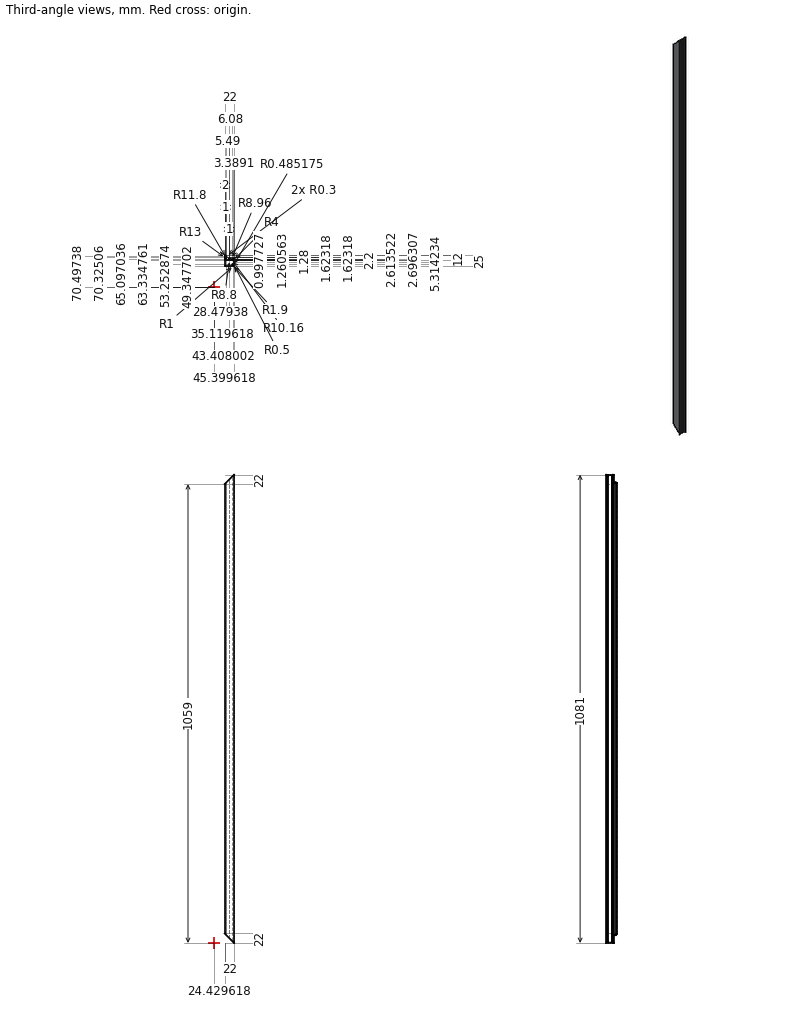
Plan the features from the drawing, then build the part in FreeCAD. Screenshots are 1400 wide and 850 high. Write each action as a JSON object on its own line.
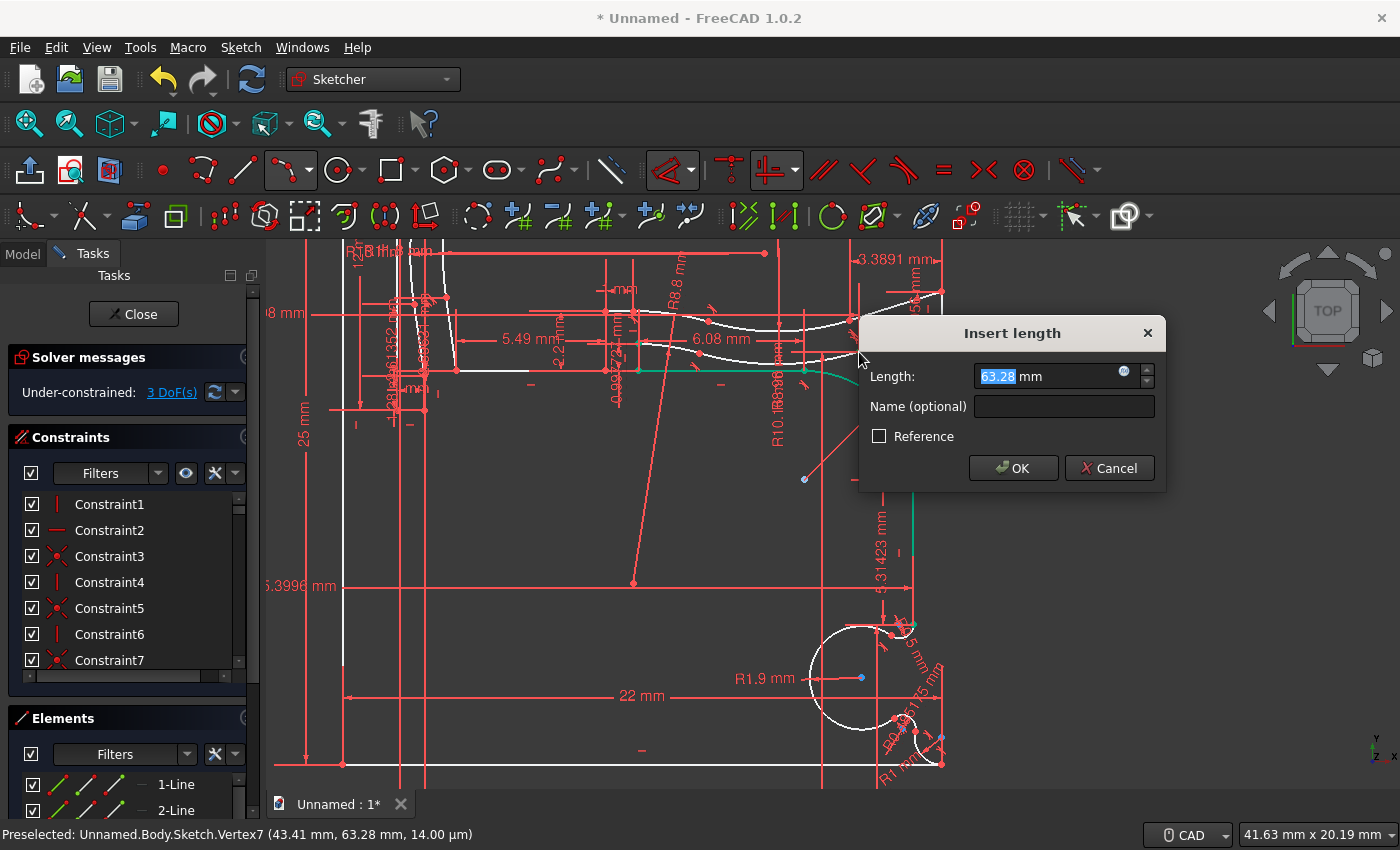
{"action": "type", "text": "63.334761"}
{"action": "key", "text": "Return"}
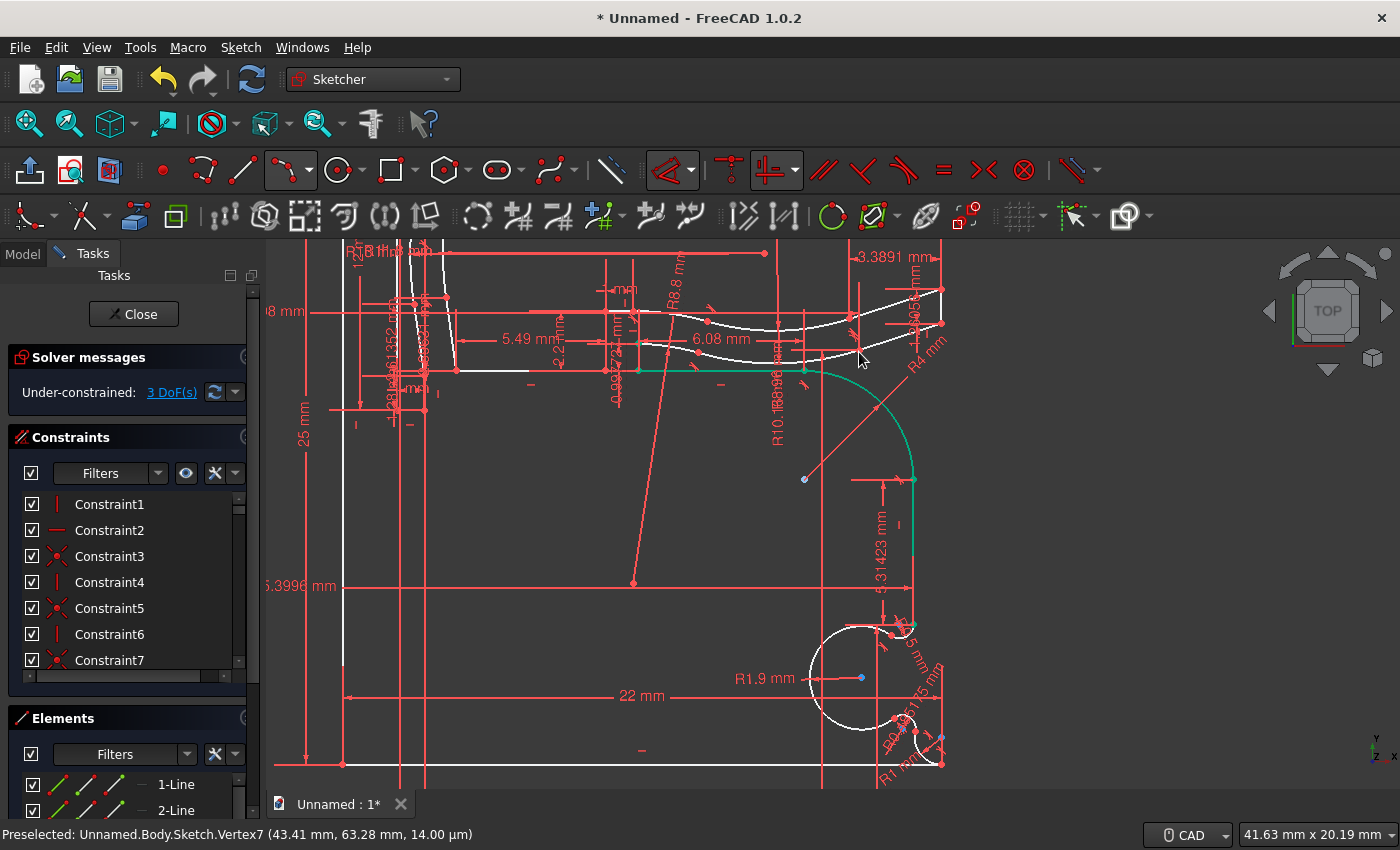
{"action": "left_click", "coordinate": [633, 311]}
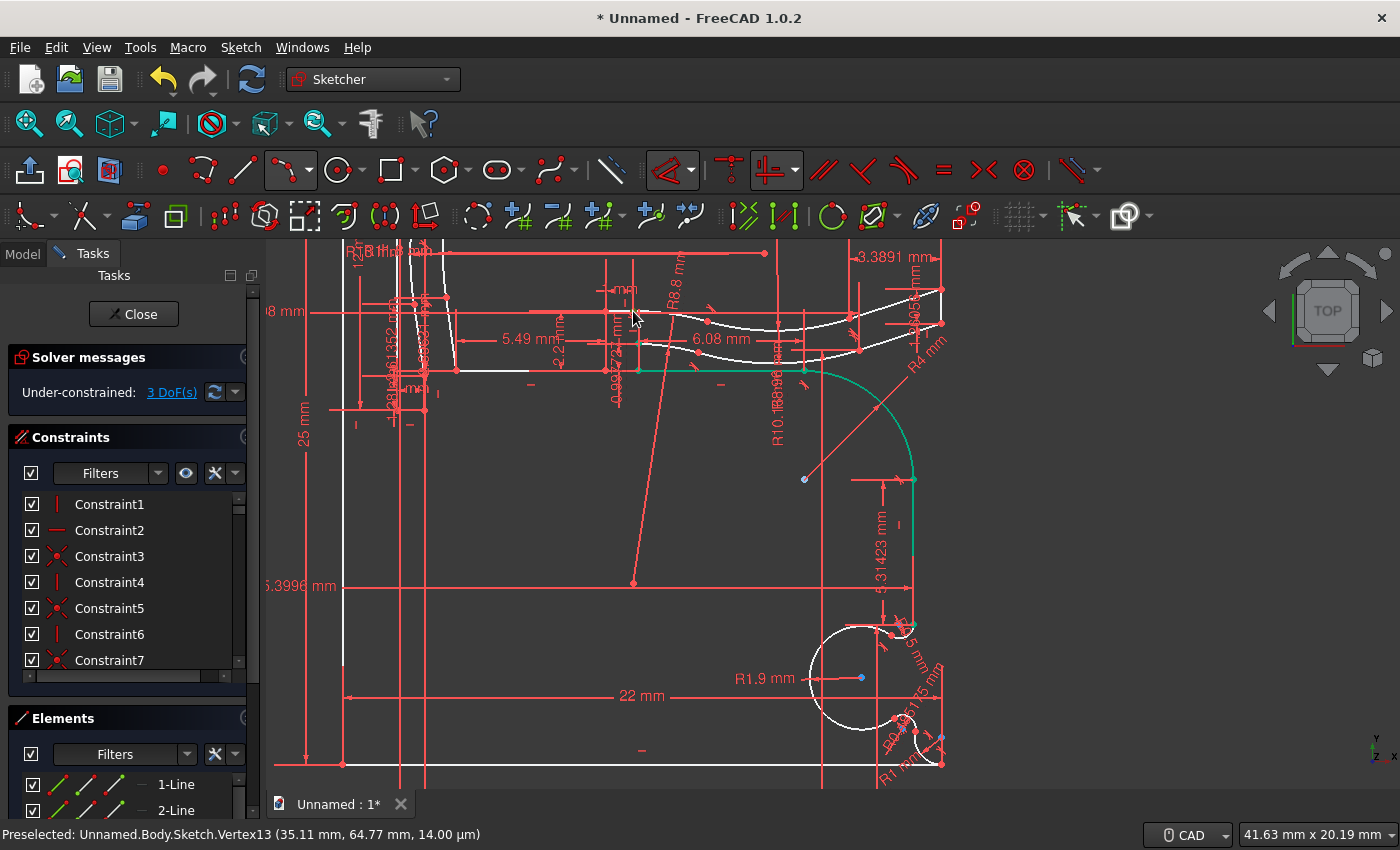
{"action": "left_click", "coordinate": [694, 170]}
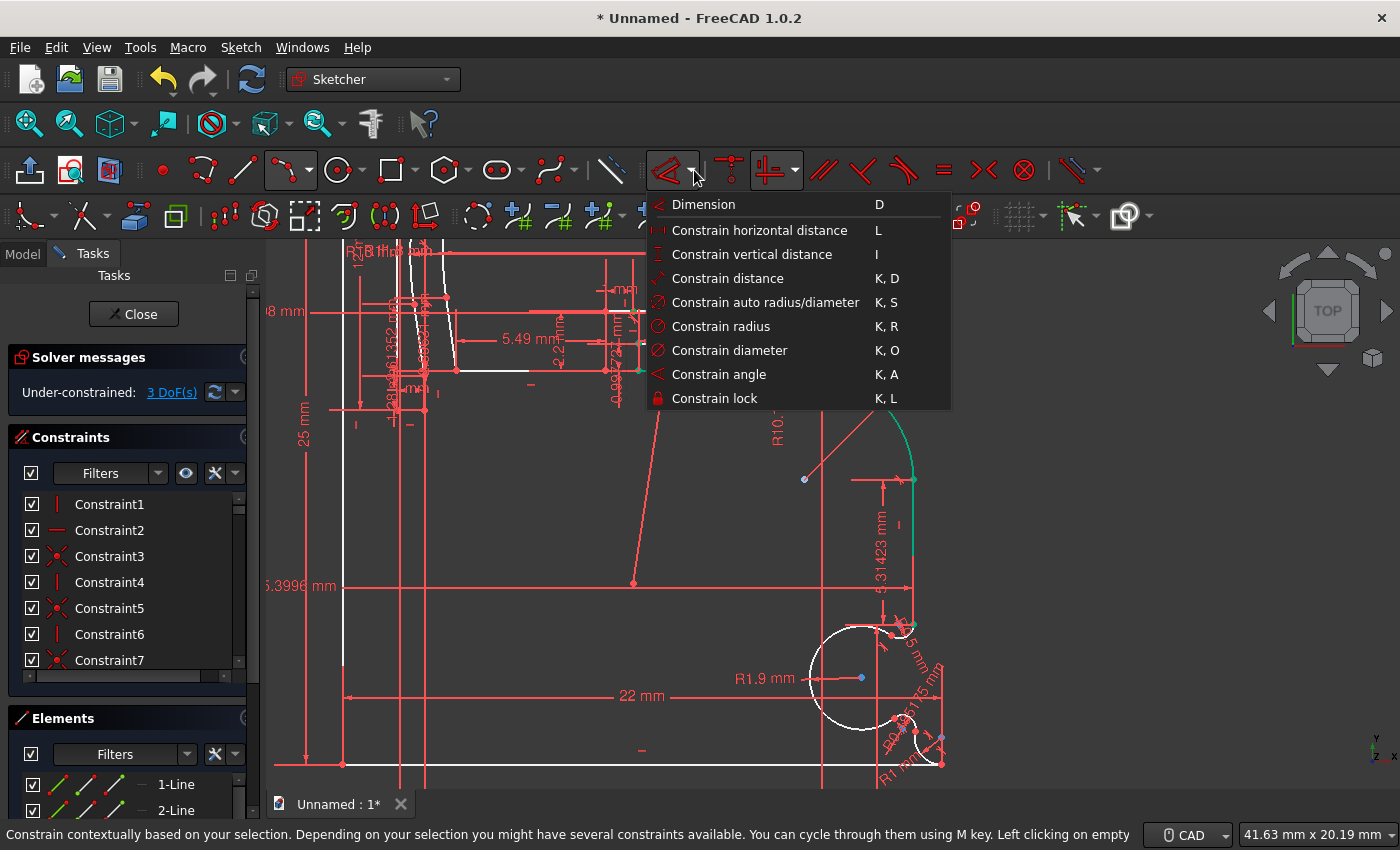
{"action": "left_click", "coordinate": [799, 230]}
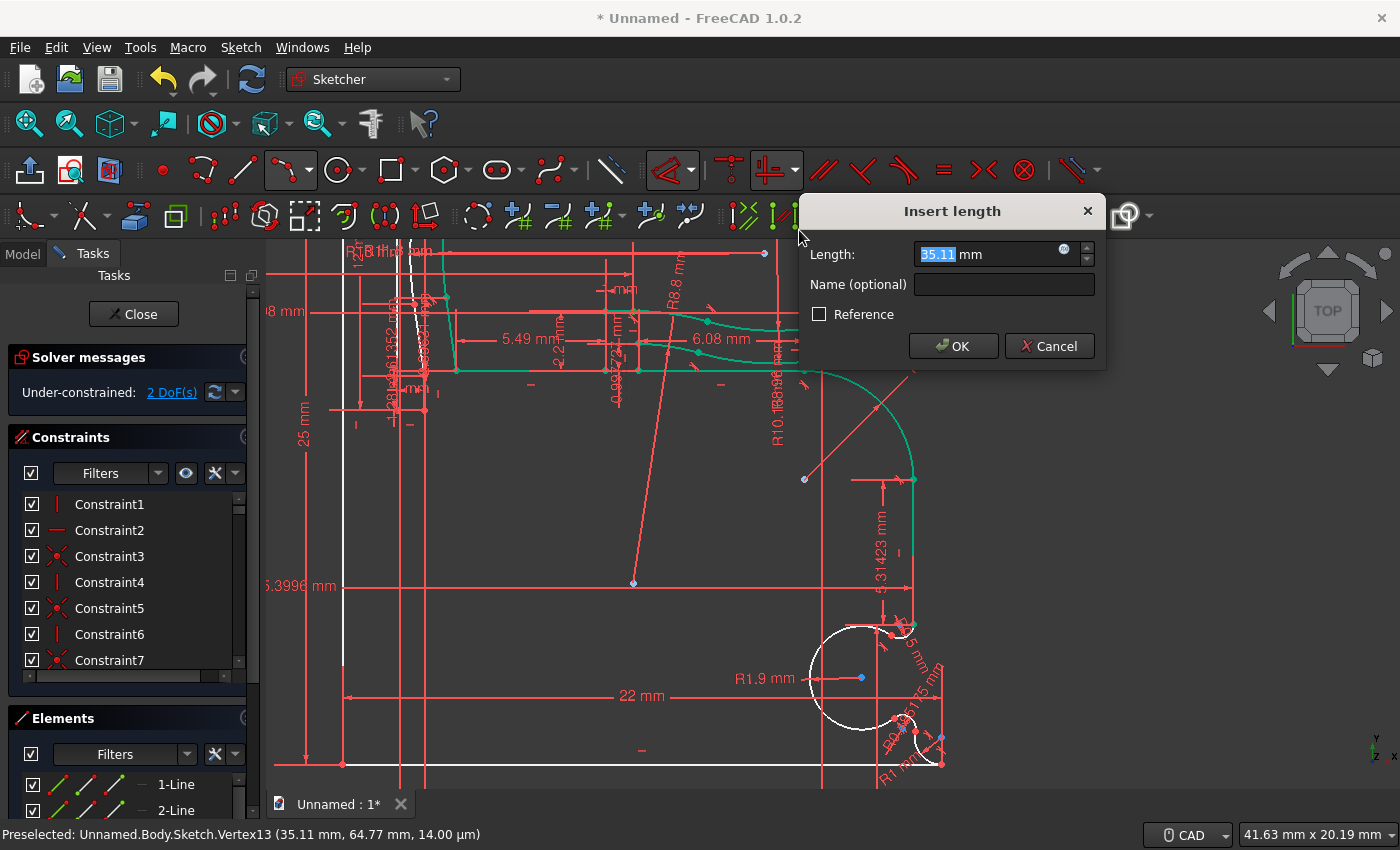
{"action": "type", "text": "35.119618"}
{"action": "key", "text": "Return"}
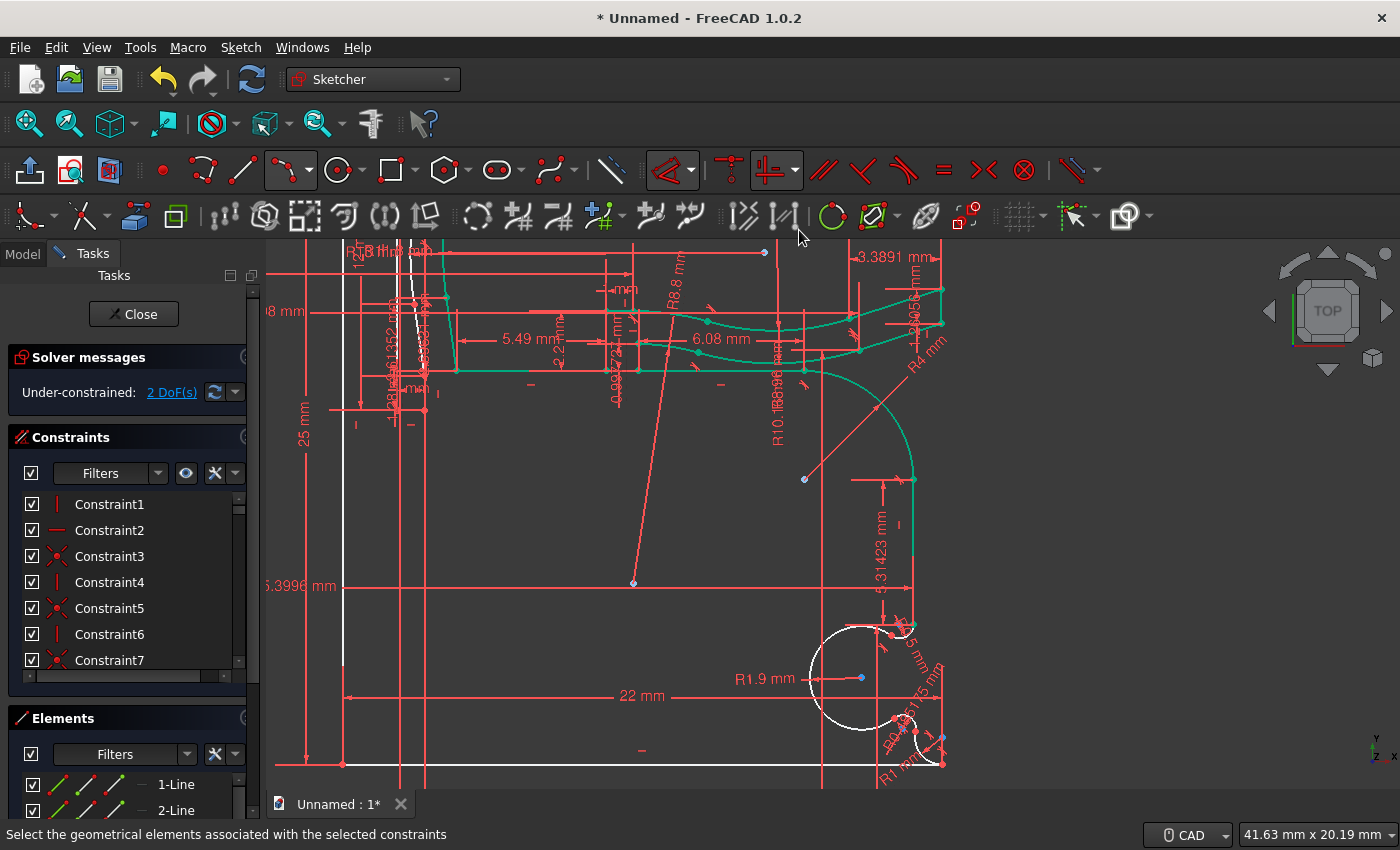
{"action": "left_click", "coordinate": [414, 304]}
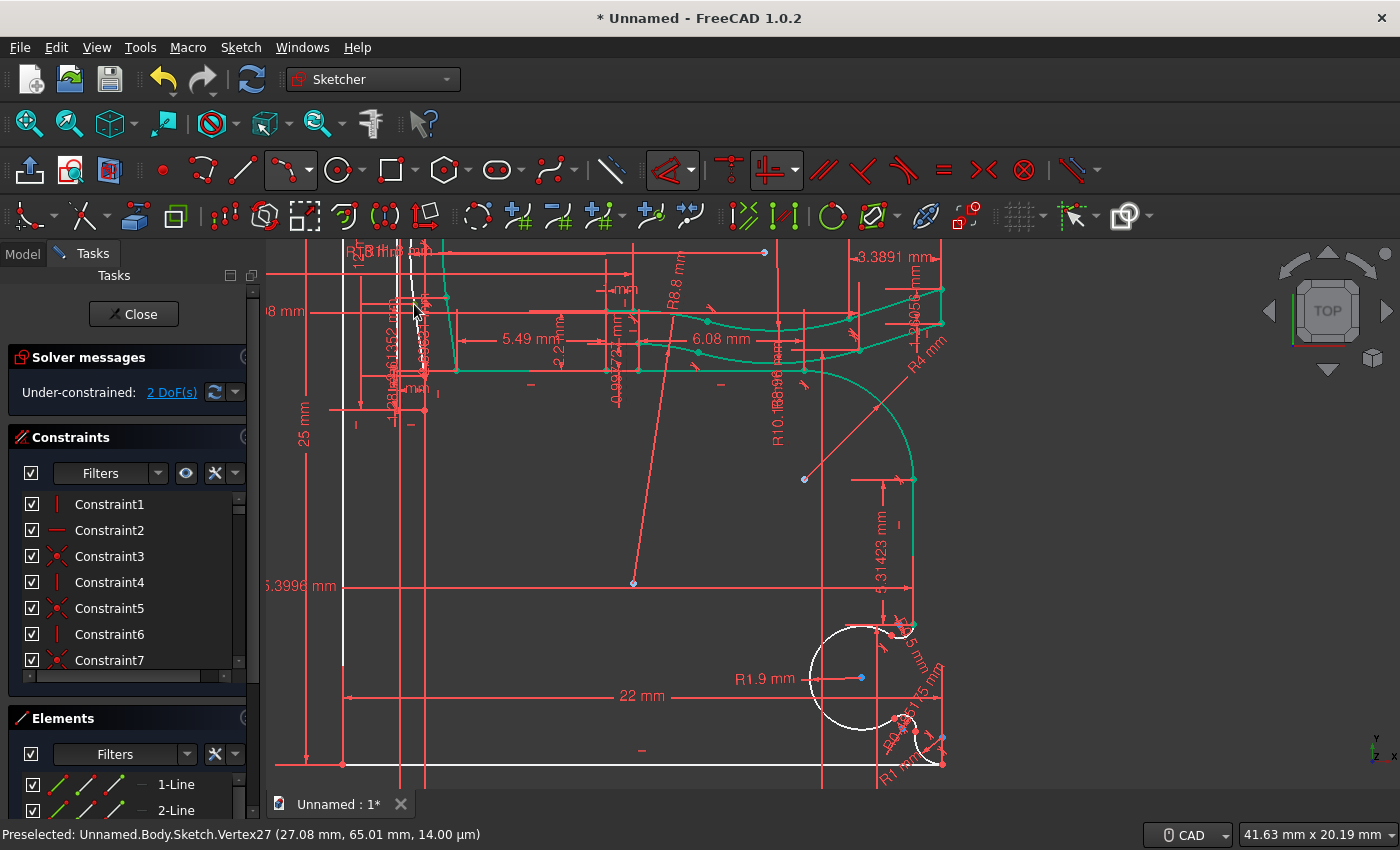
{"action": "key", "text": "i"}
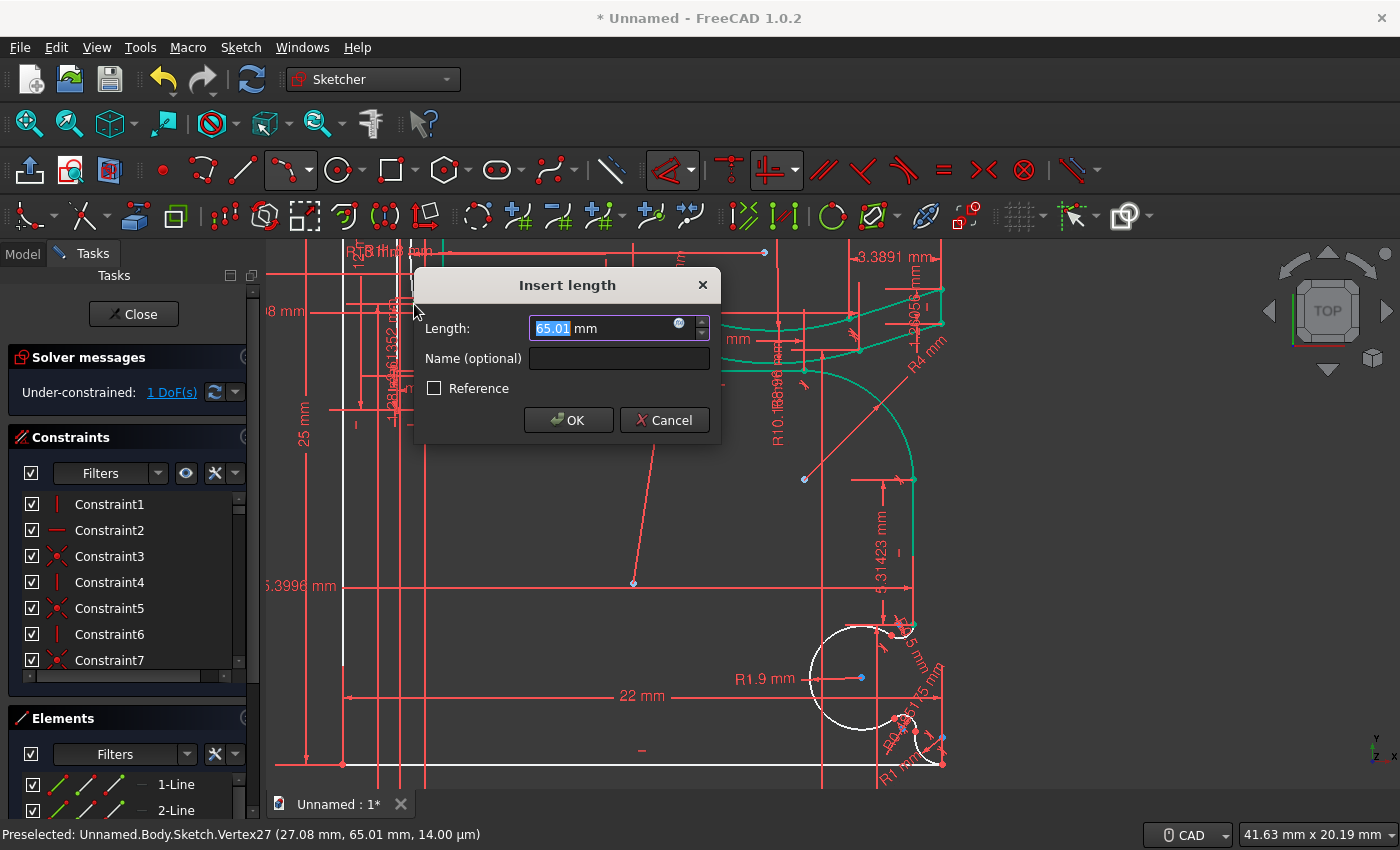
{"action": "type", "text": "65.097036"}
{"action": "key", "text": "Return"}